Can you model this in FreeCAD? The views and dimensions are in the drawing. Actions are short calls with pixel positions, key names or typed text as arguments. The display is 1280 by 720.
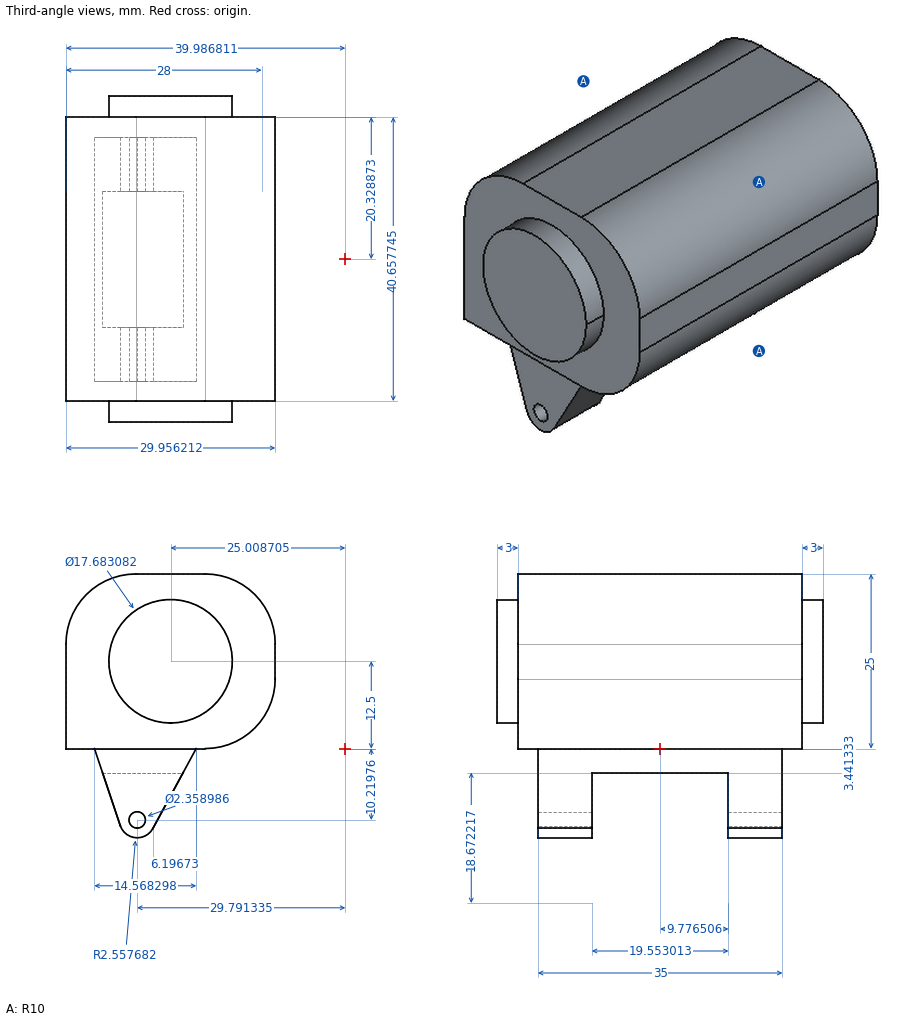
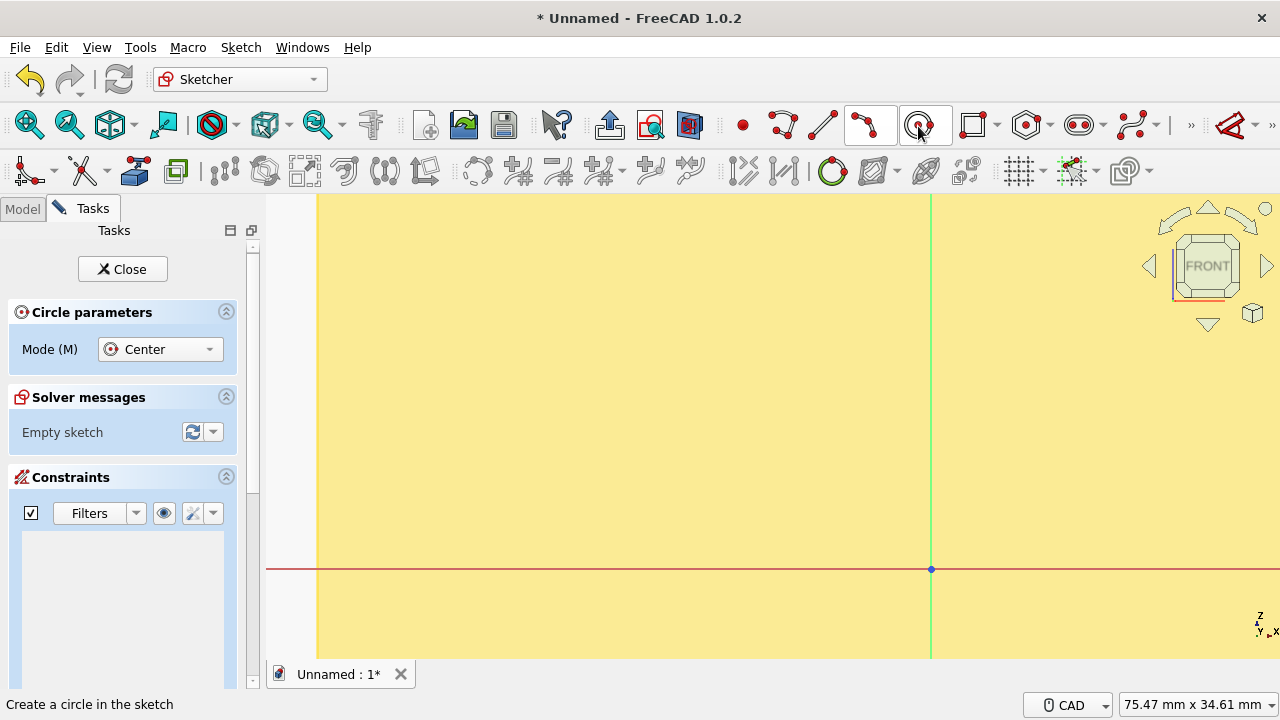
click(595, 401)
move(679, 317)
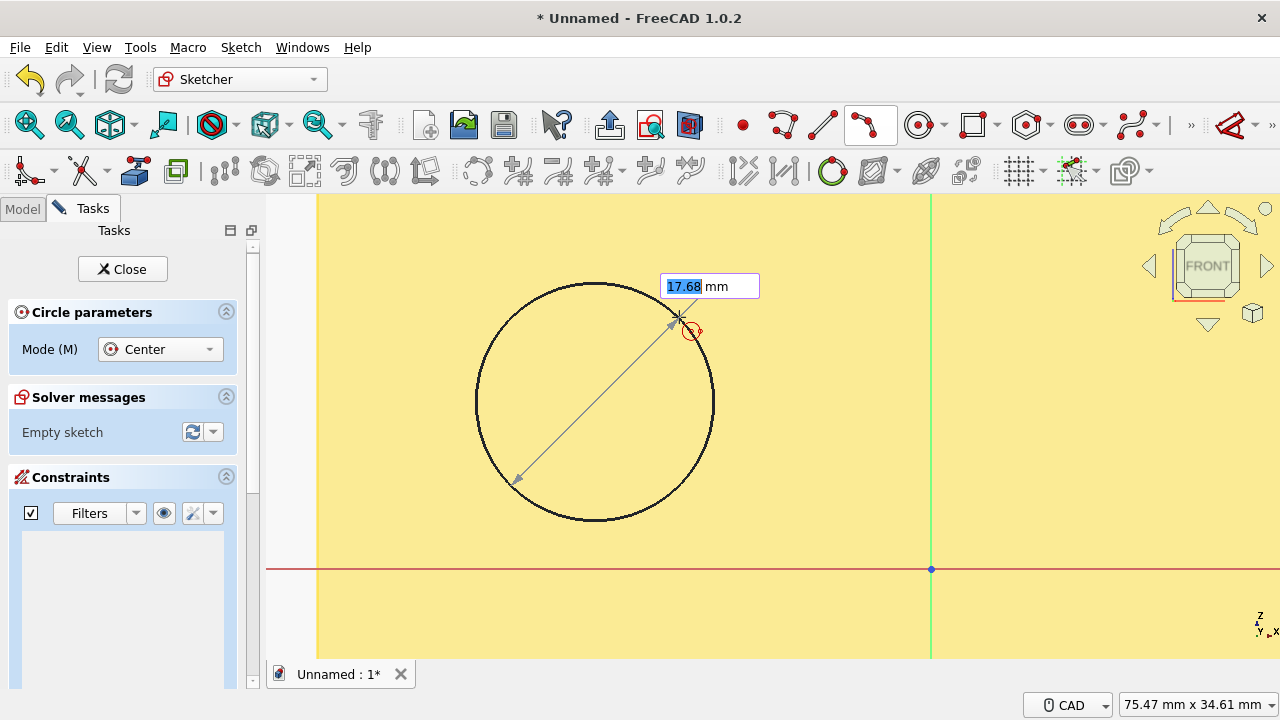
text(17.683082)
key(Return)
key(Escape)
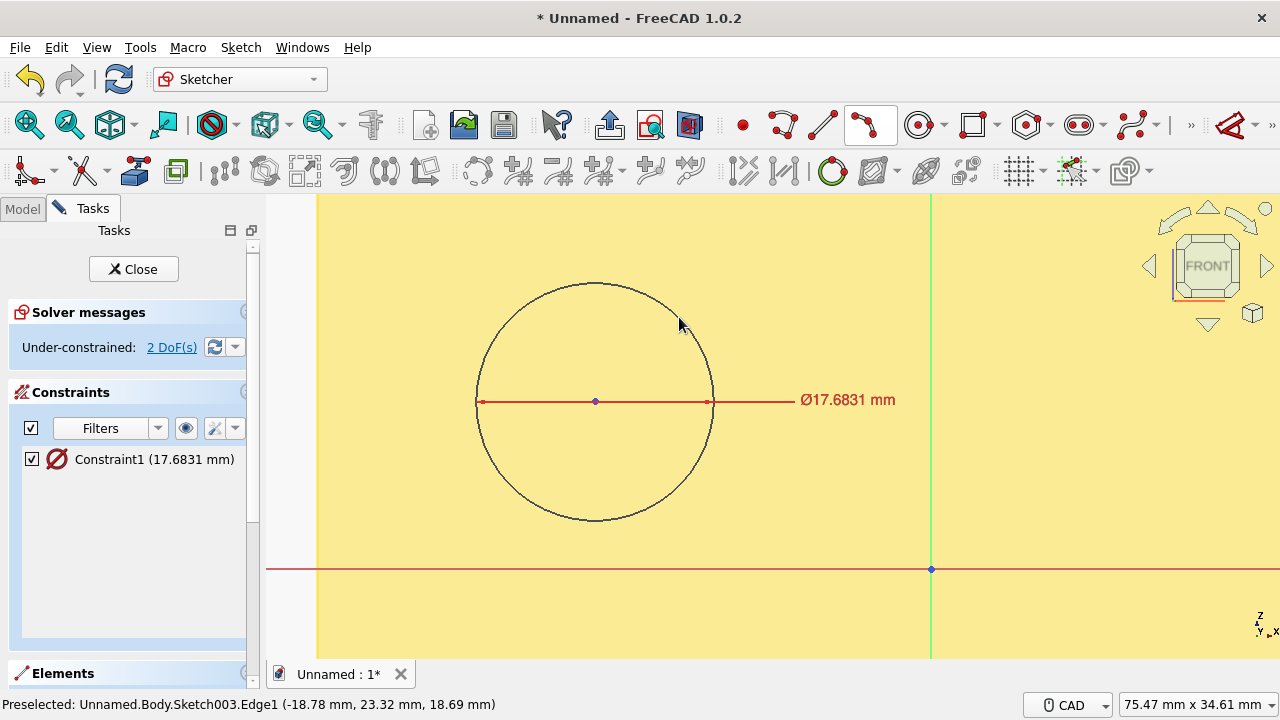
click(1230, 126)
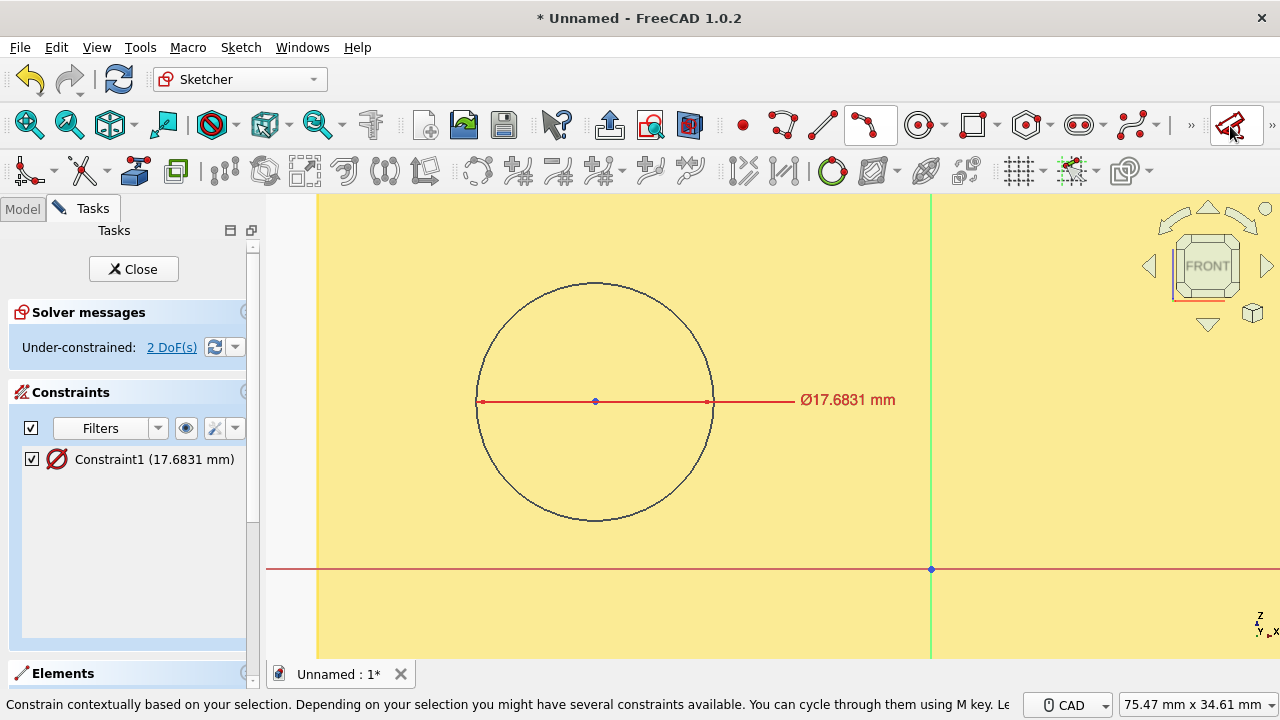
click(595, 402)
click(965, 486)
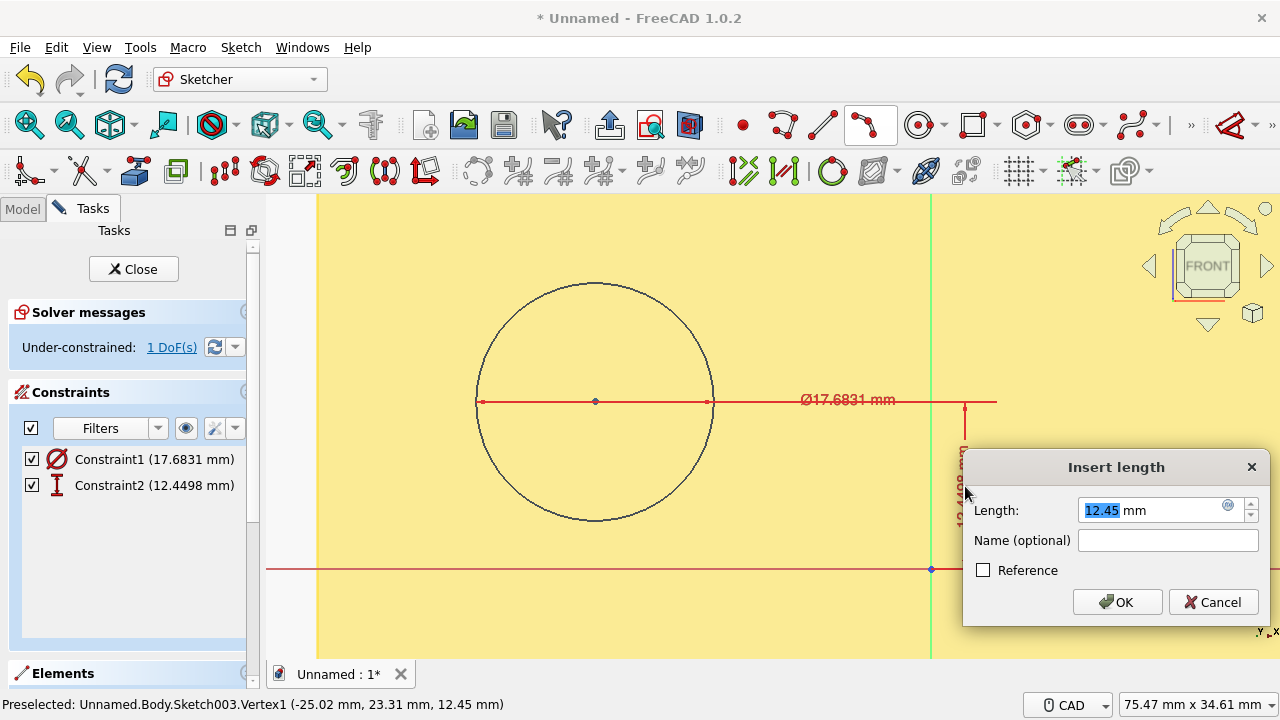
text(12.5)
key(Return)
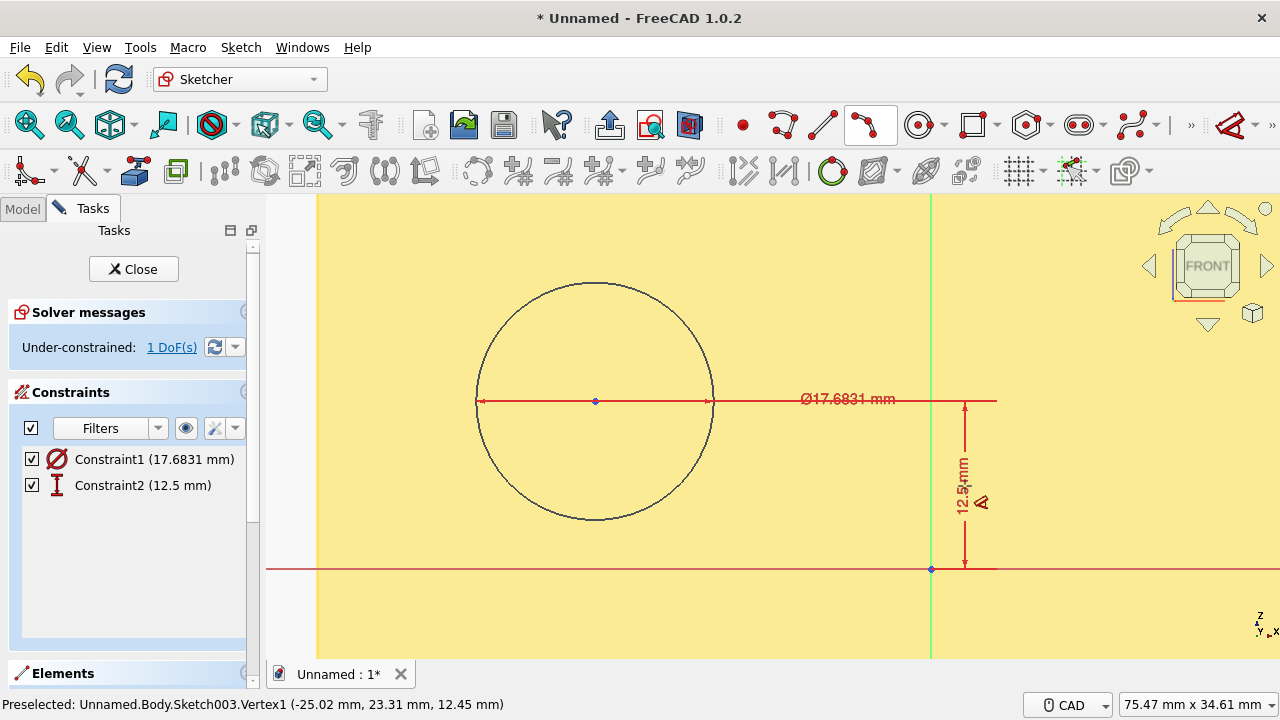
click(595, 401)
click(763, 603)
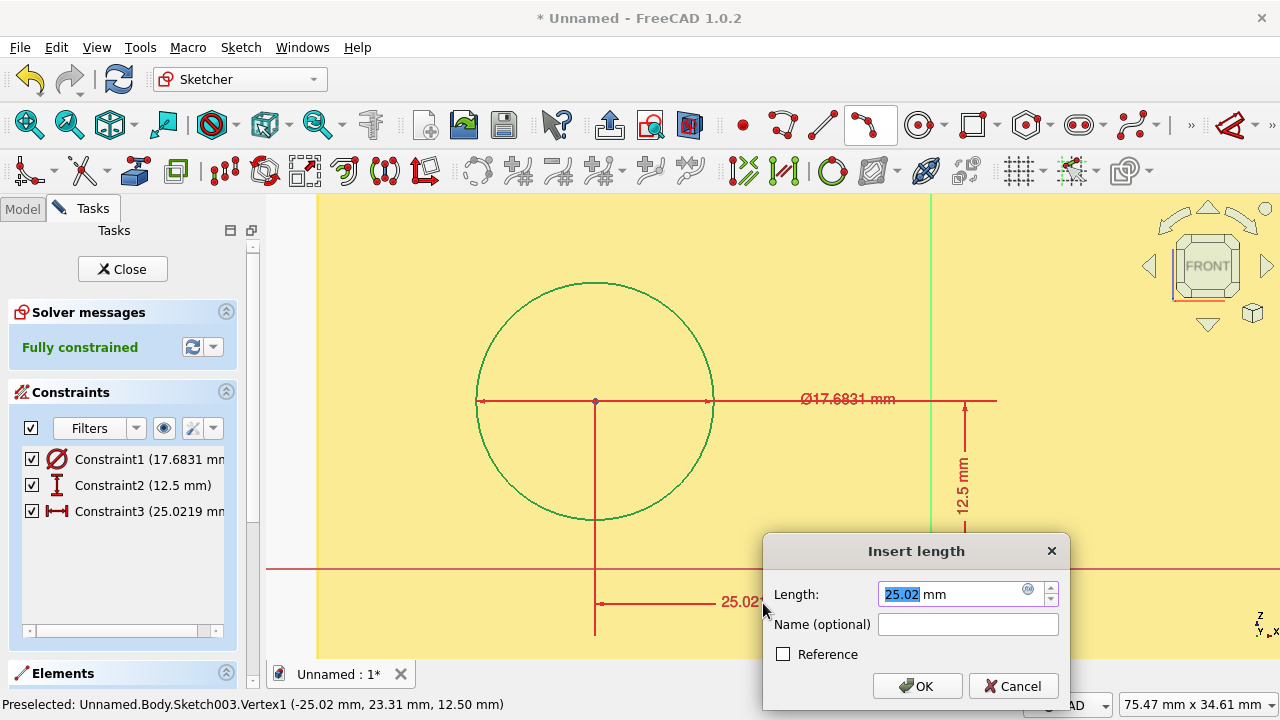
text(25.008705)
key(Return)
key(Escape)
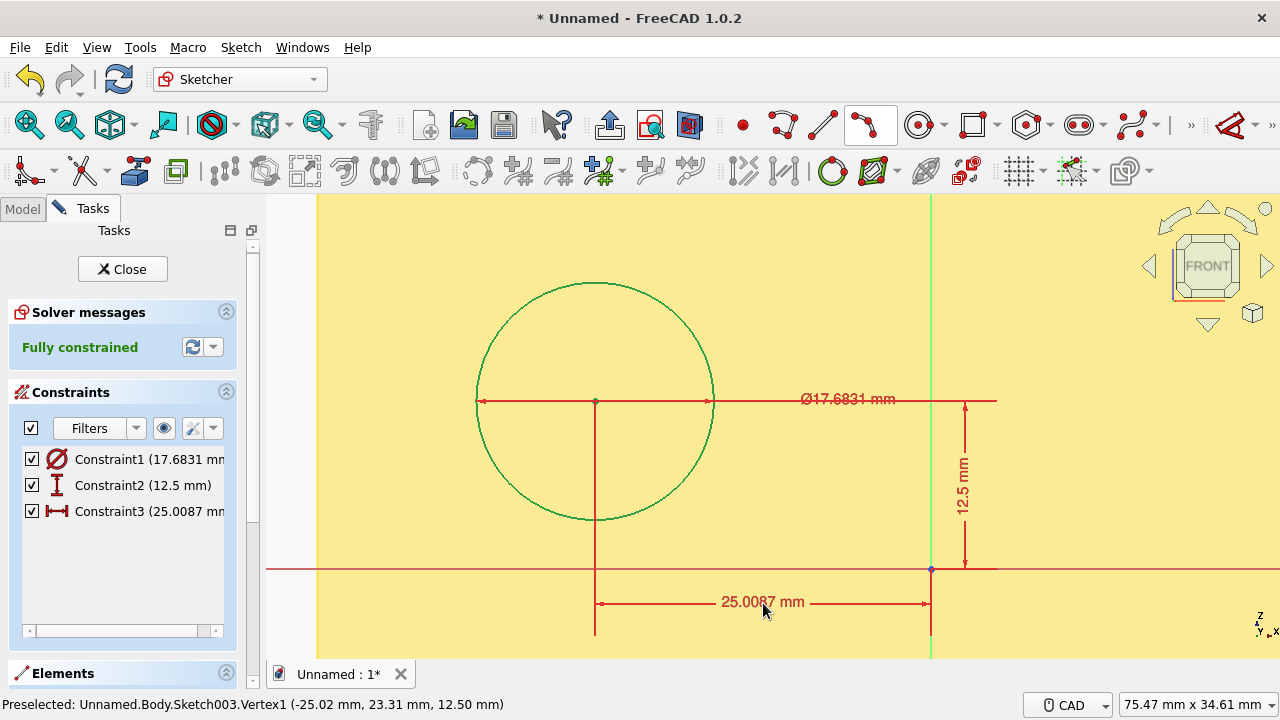
click(123, 269)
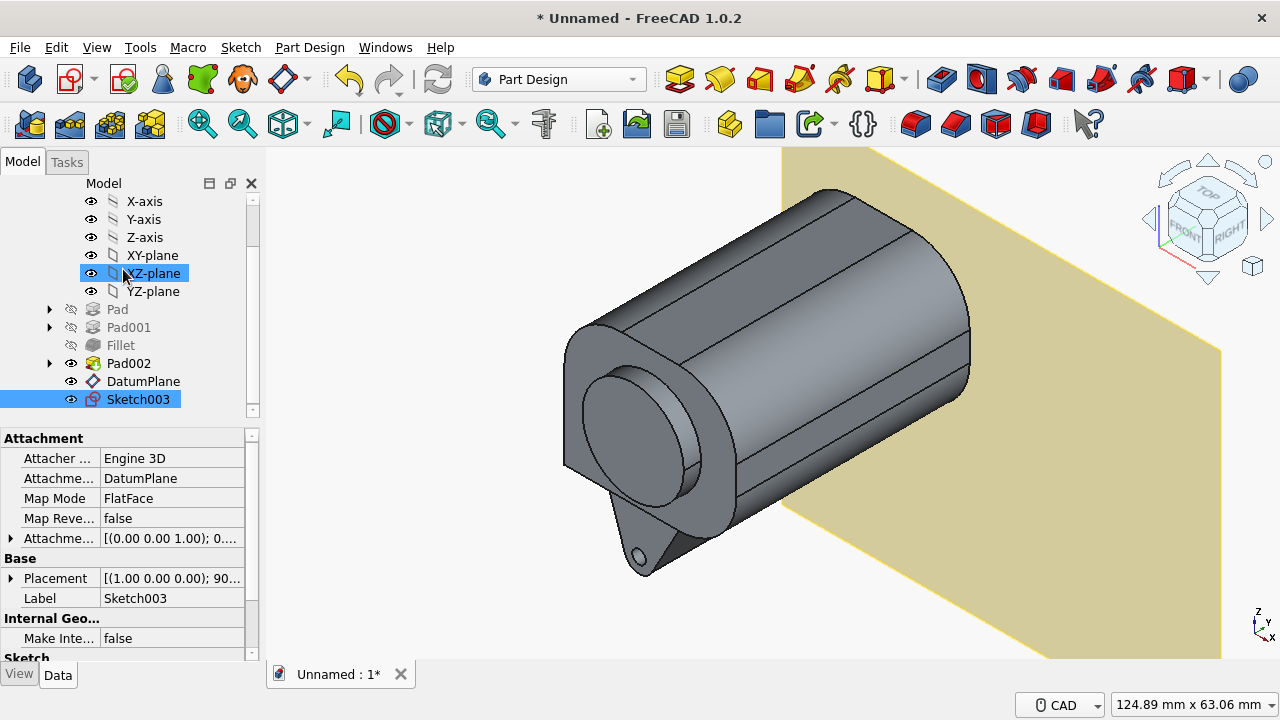
click(680, 80)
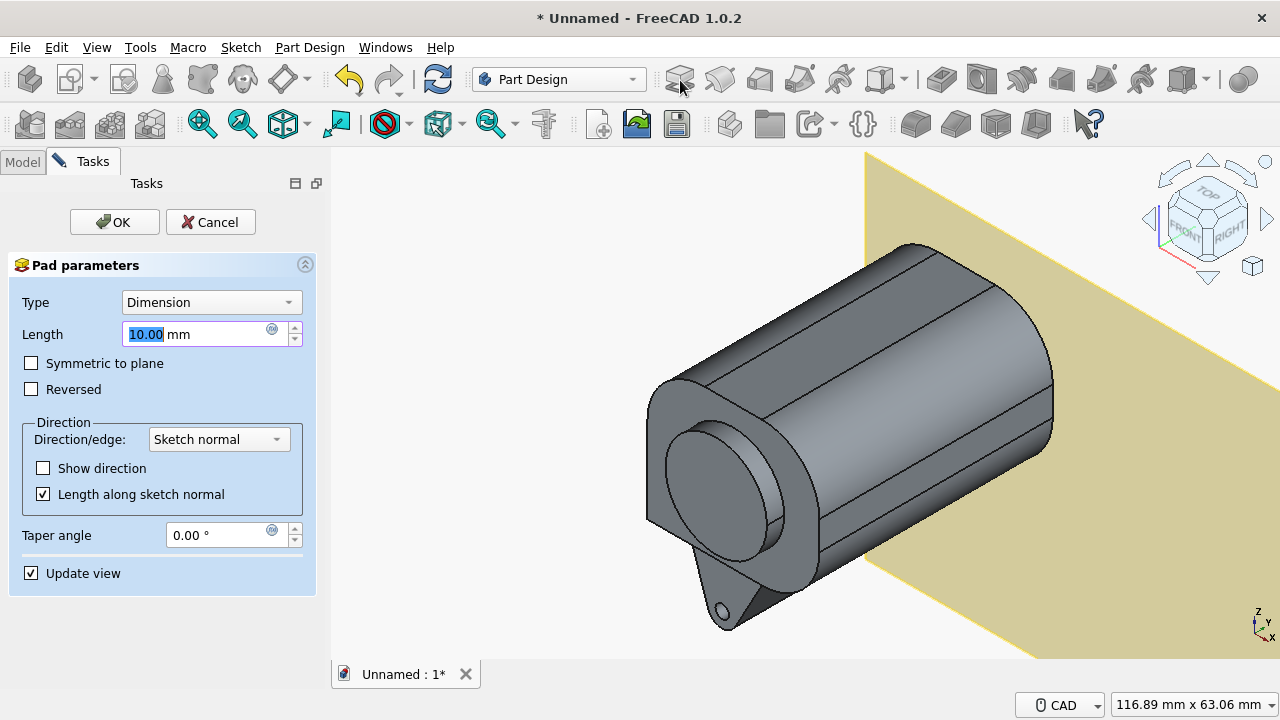
text(3)
key(Tab)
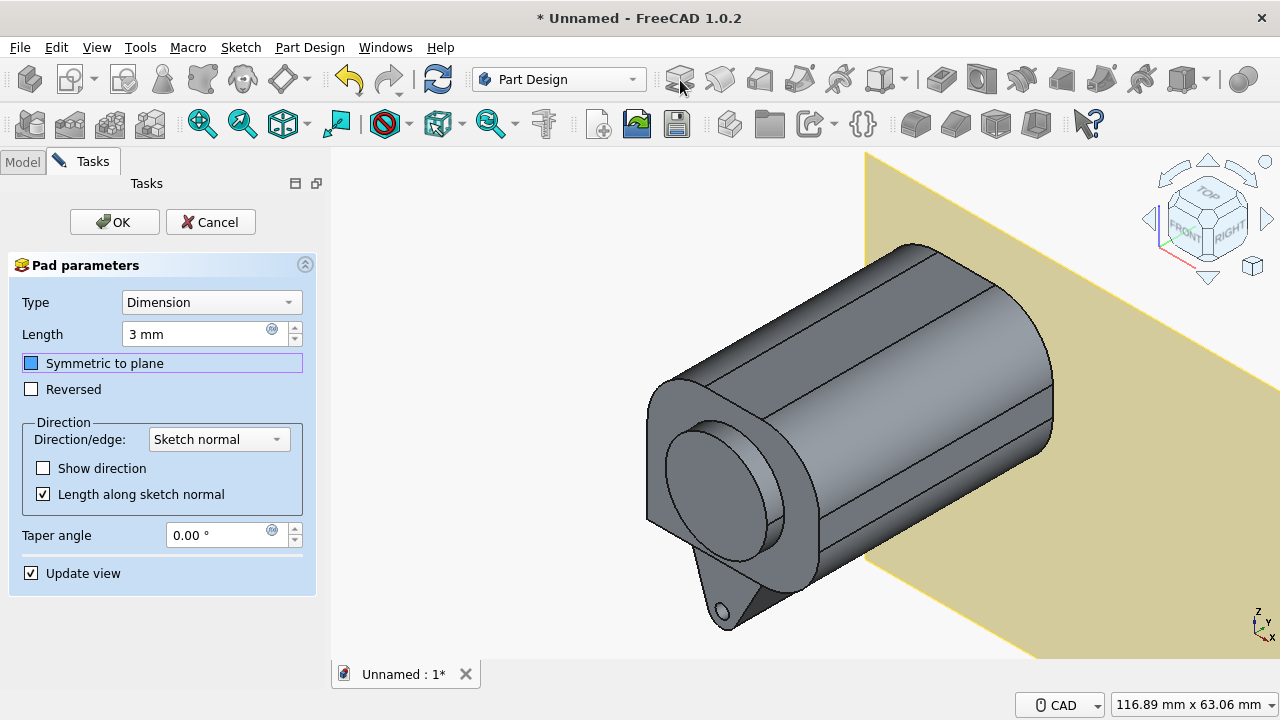
click(115, 222)